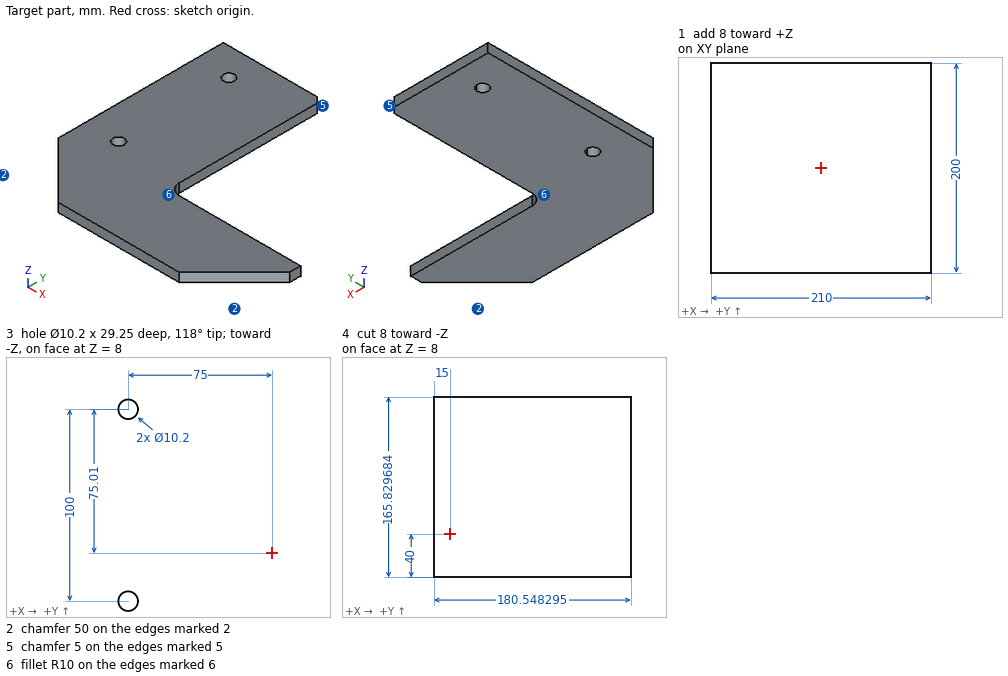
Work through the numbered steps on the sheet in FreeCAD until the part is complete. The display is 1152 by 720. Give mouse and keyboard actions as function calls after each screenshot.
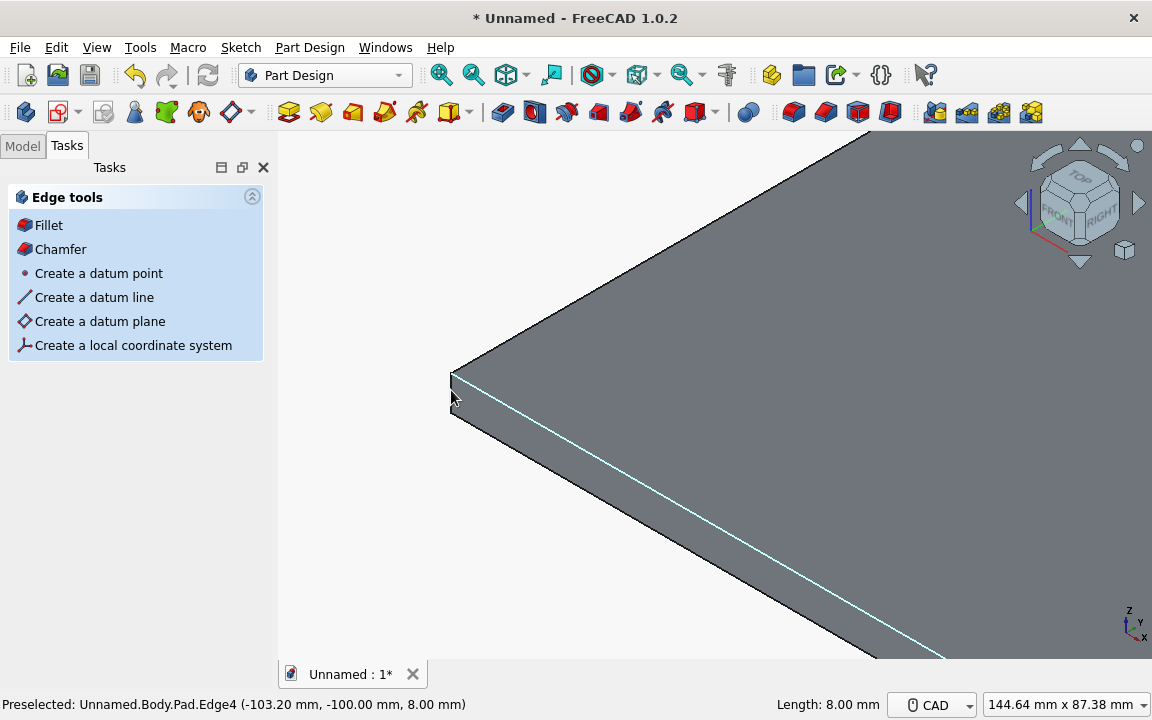
key(v)
key(f)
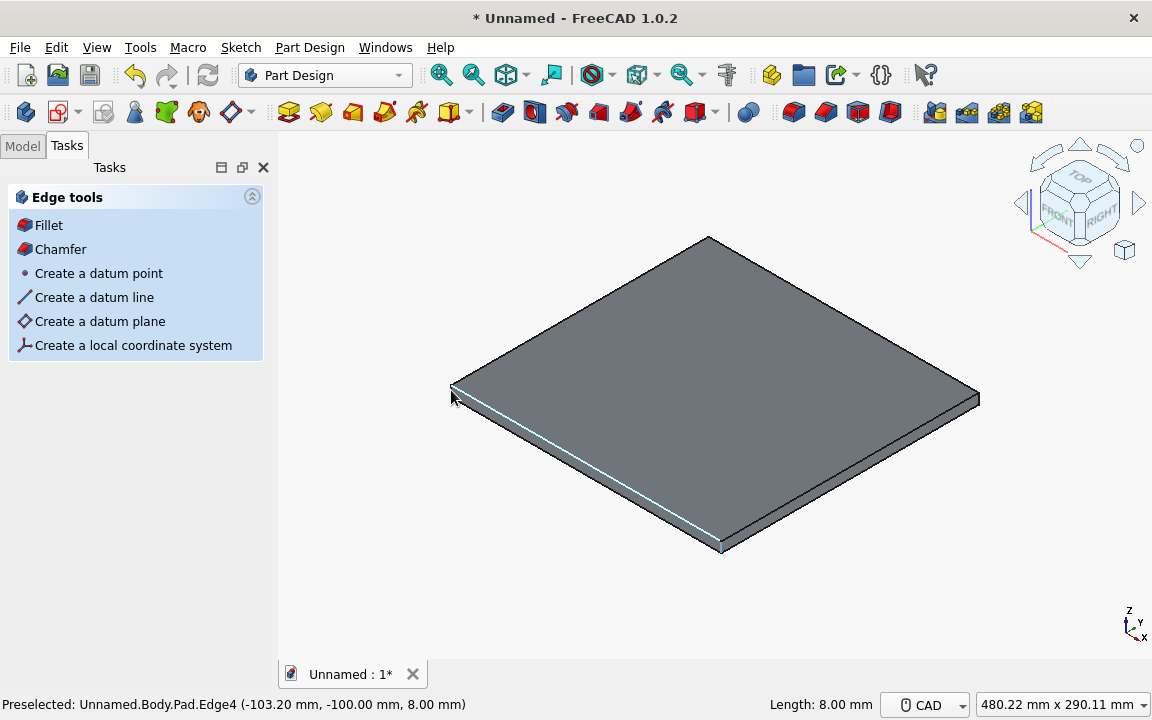
key(2)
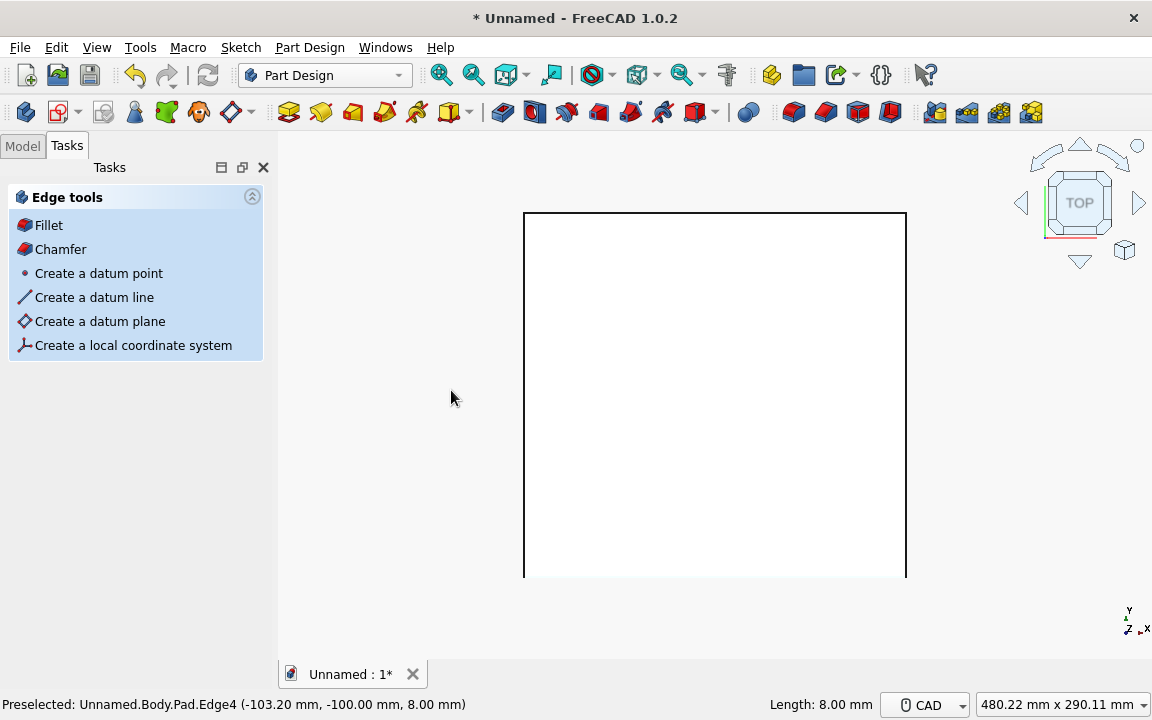
scroll(524, 576, up, 6)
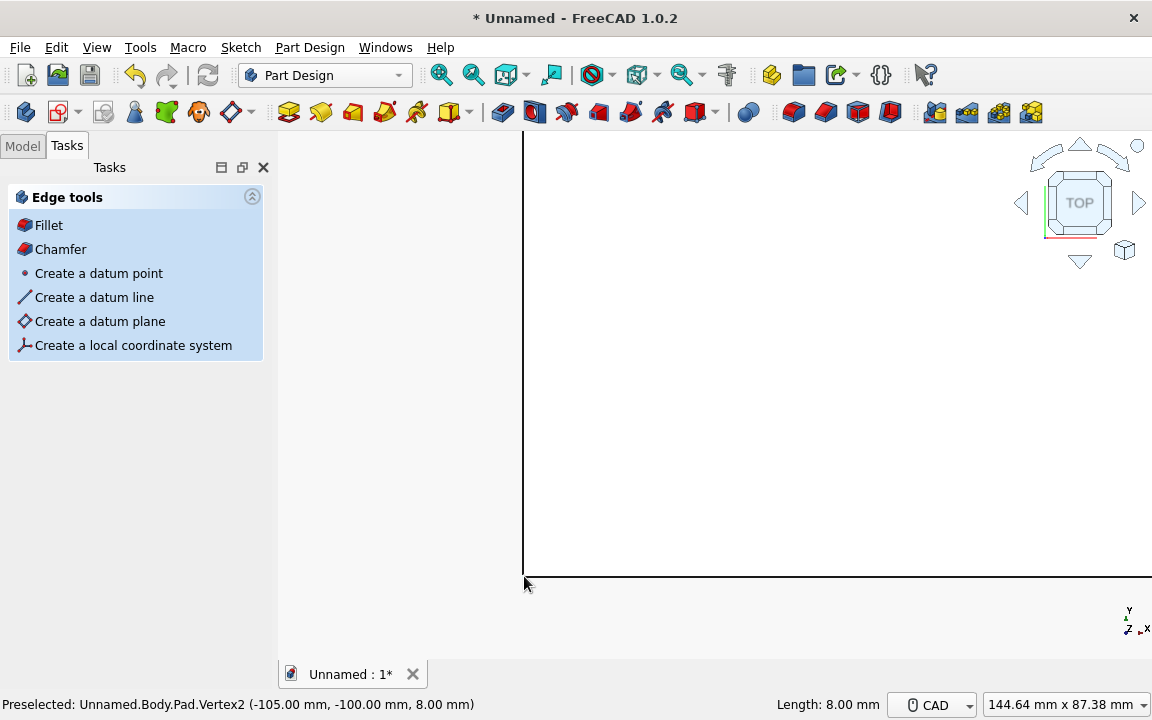
key(v)
key(f)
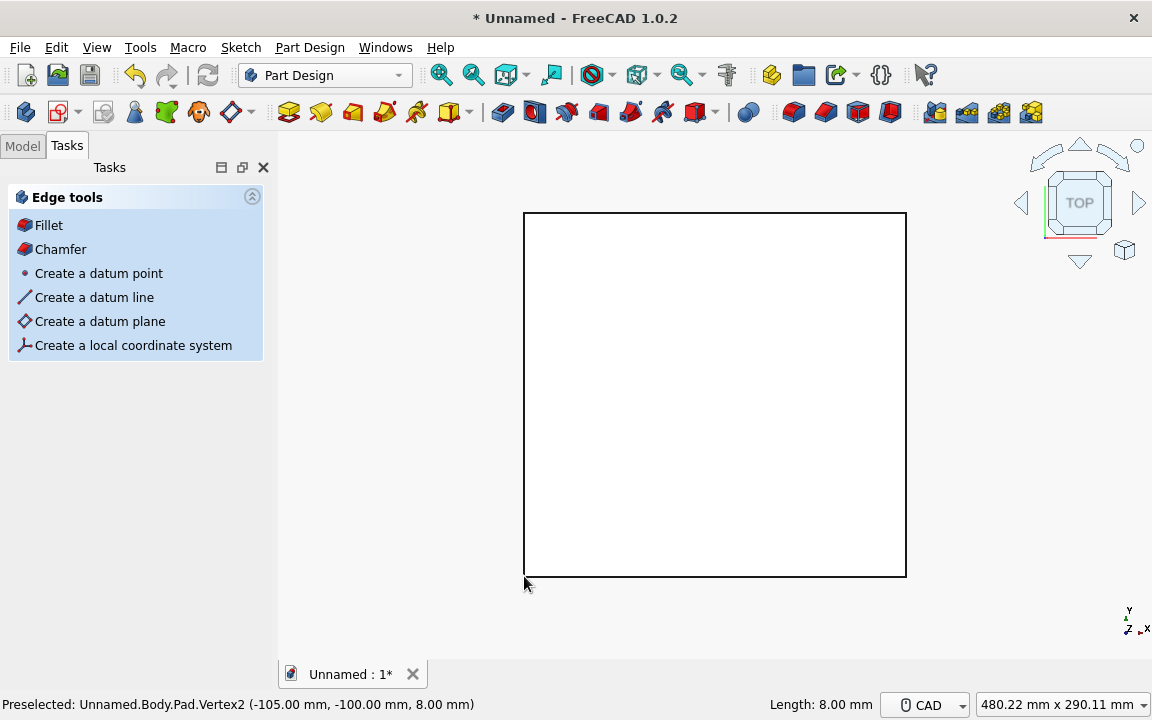
key(1)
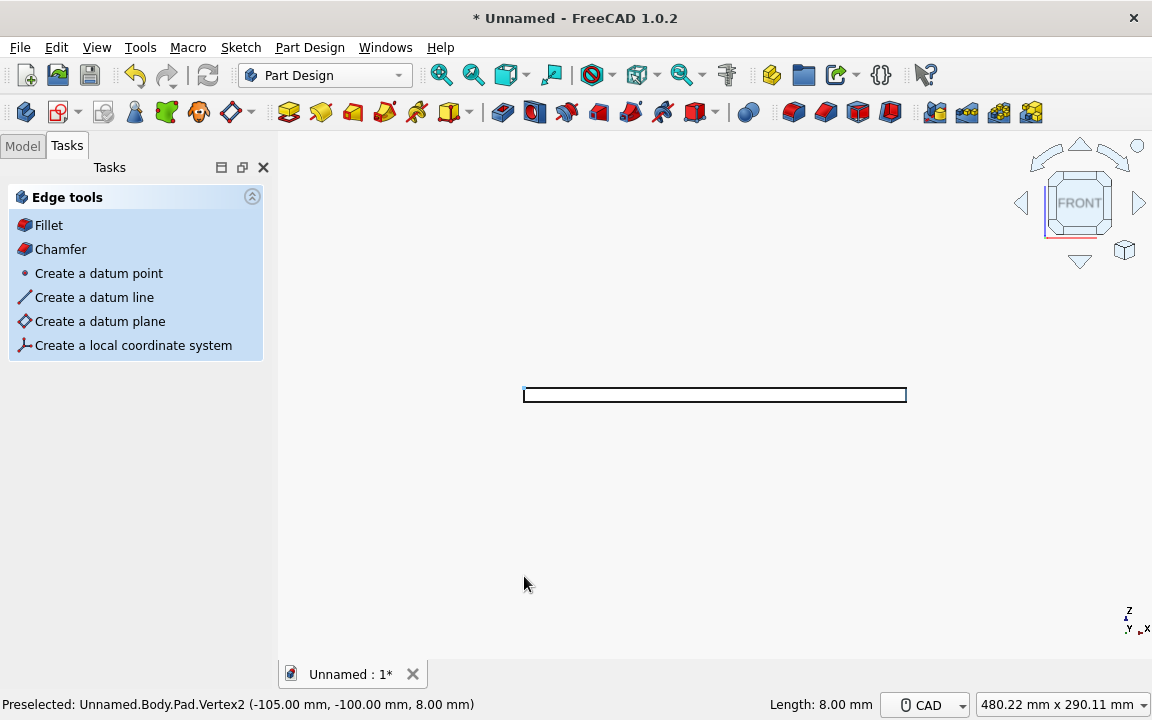
key(v)
key(f)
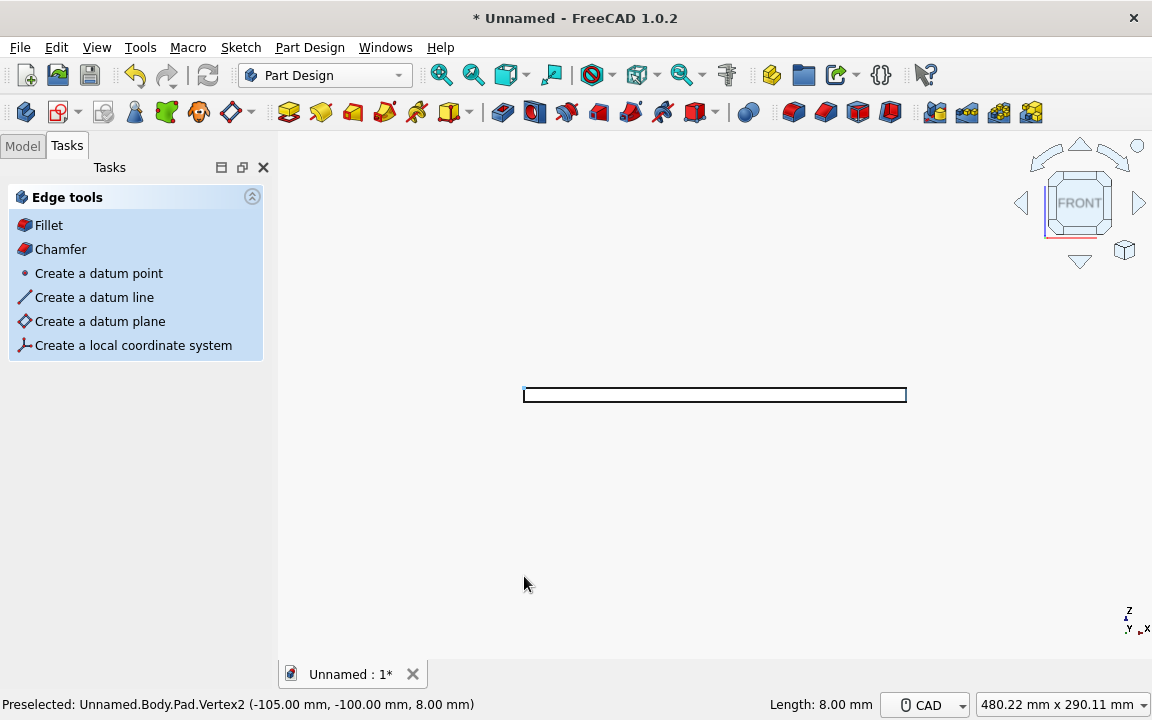
click(524, 394, ctrl)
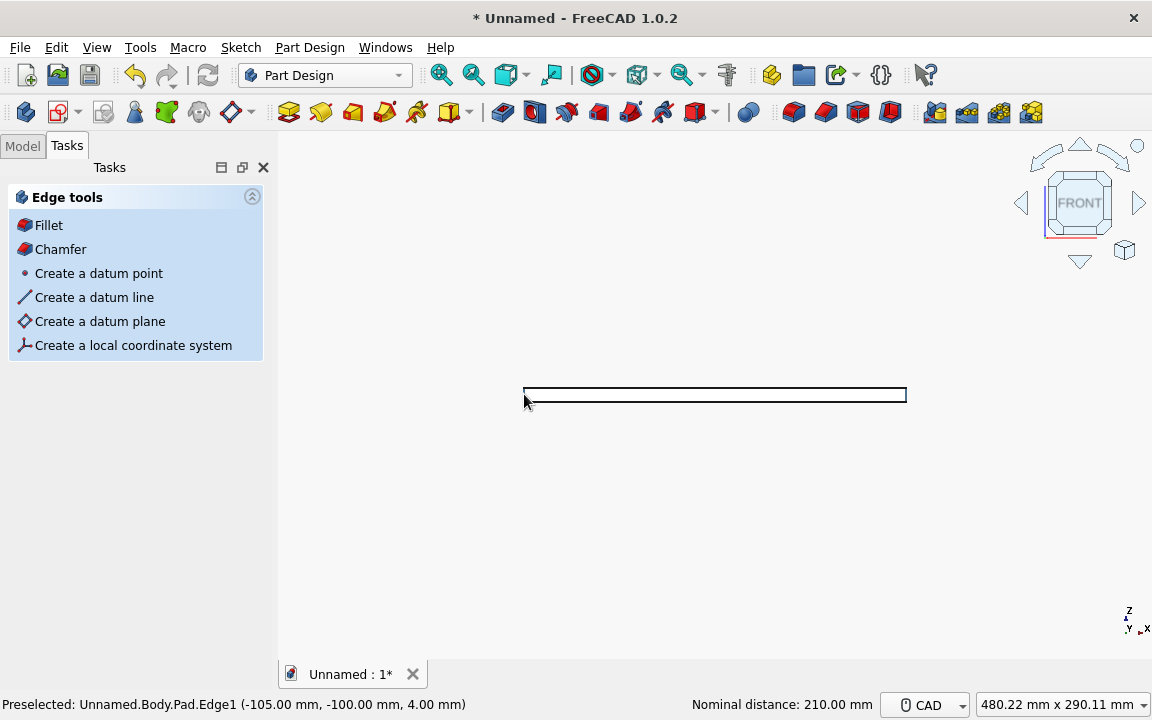
click(826, 112)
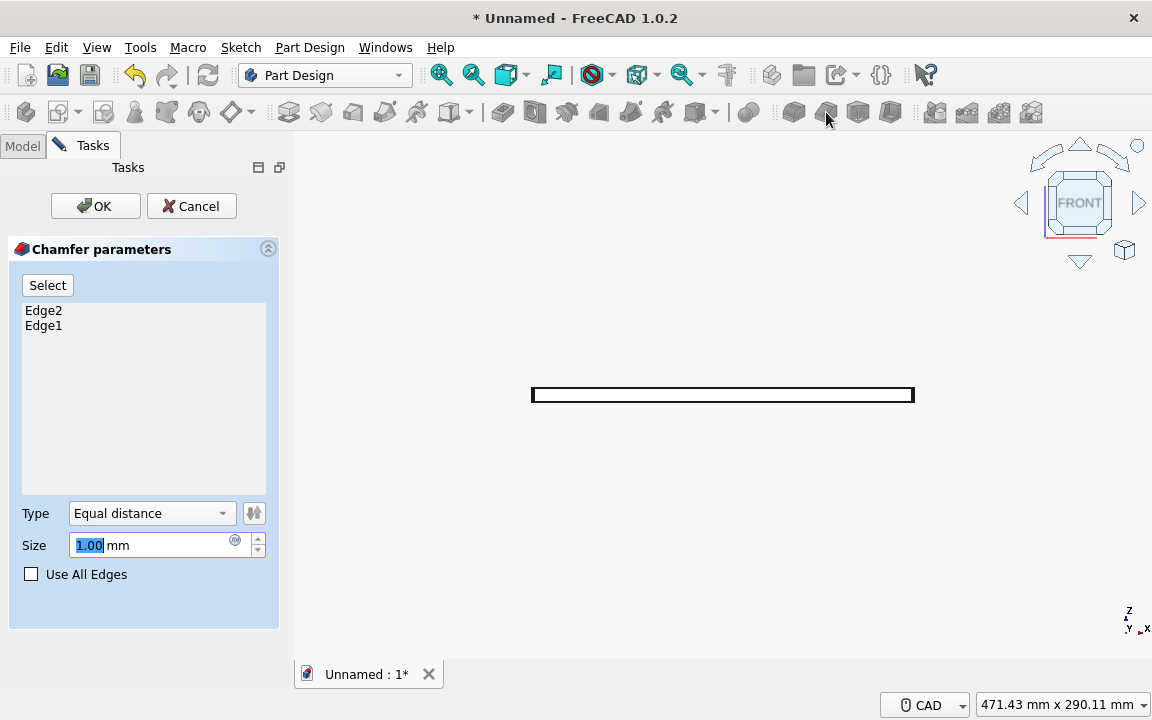
text(50)
key(Tab)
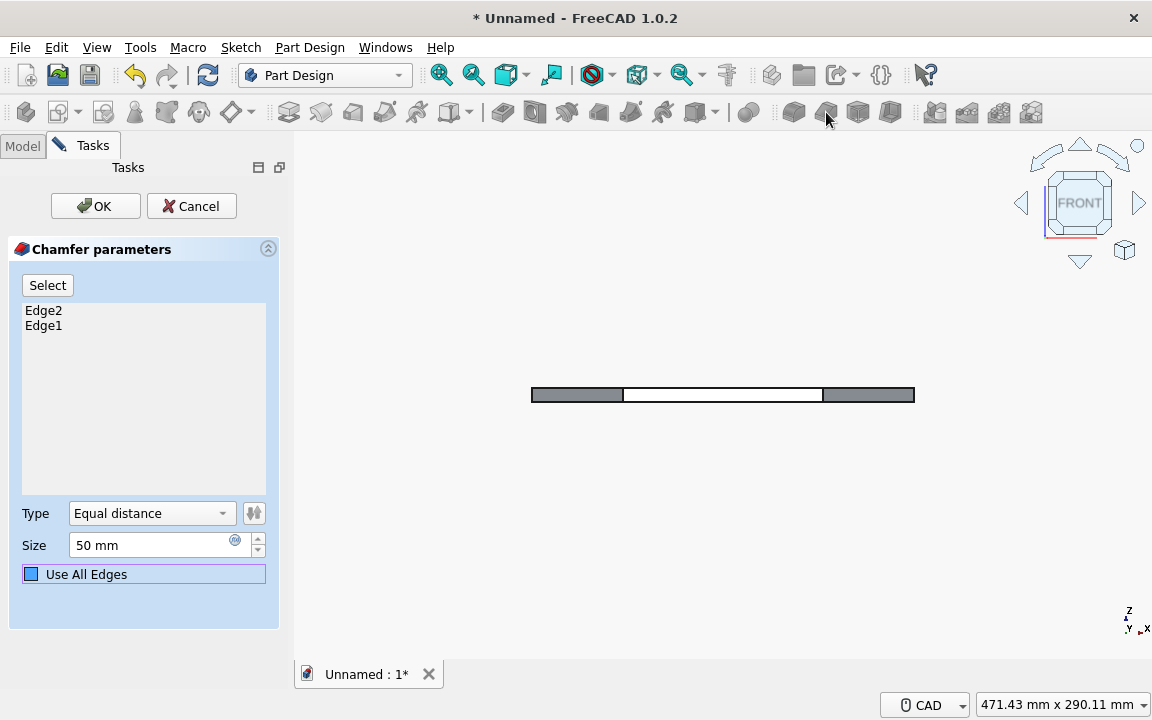
click(96, 206)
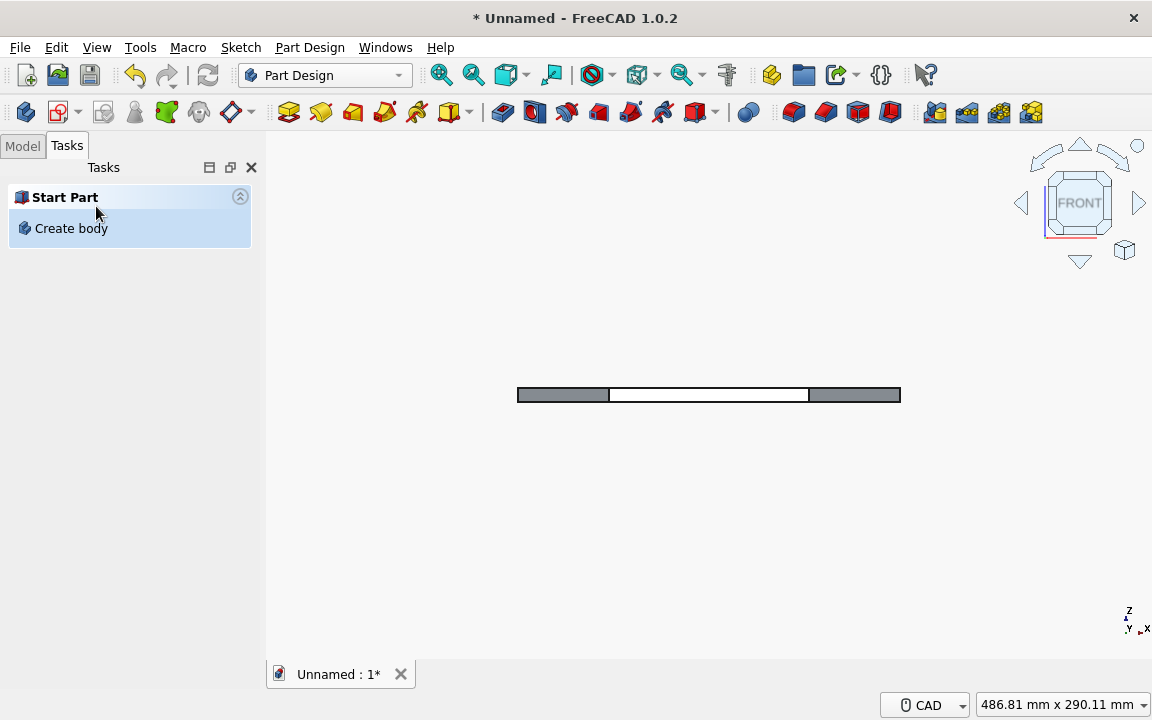
key(v)
key(f)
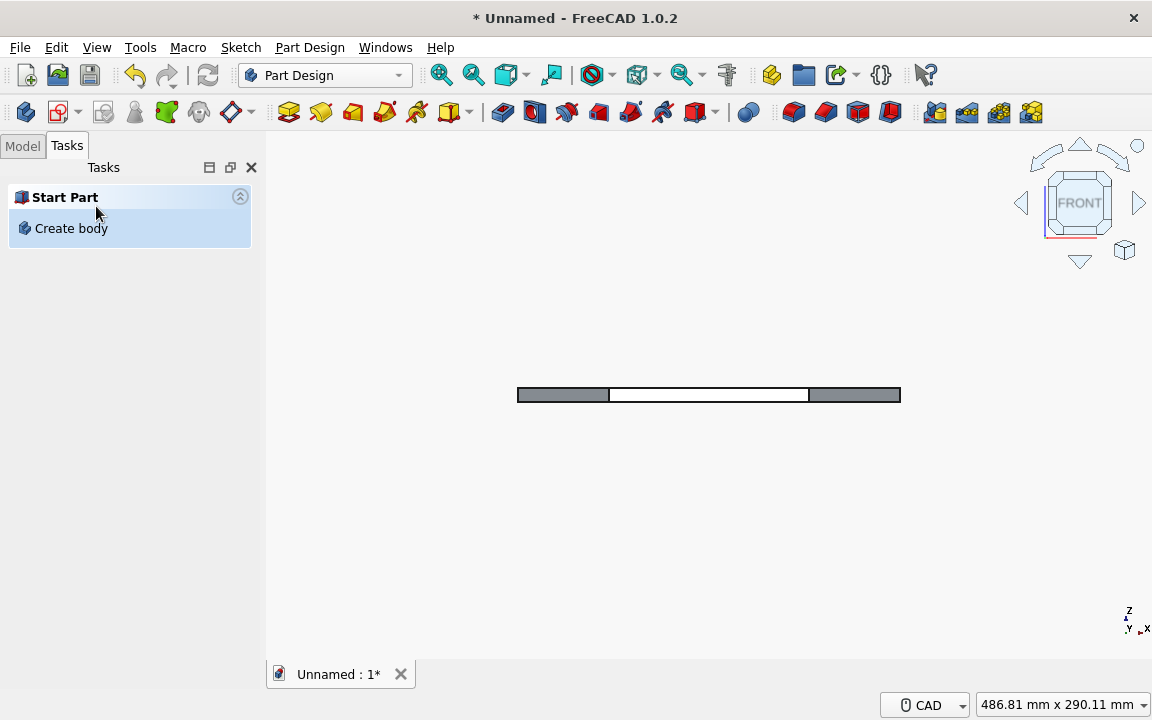
key(0)